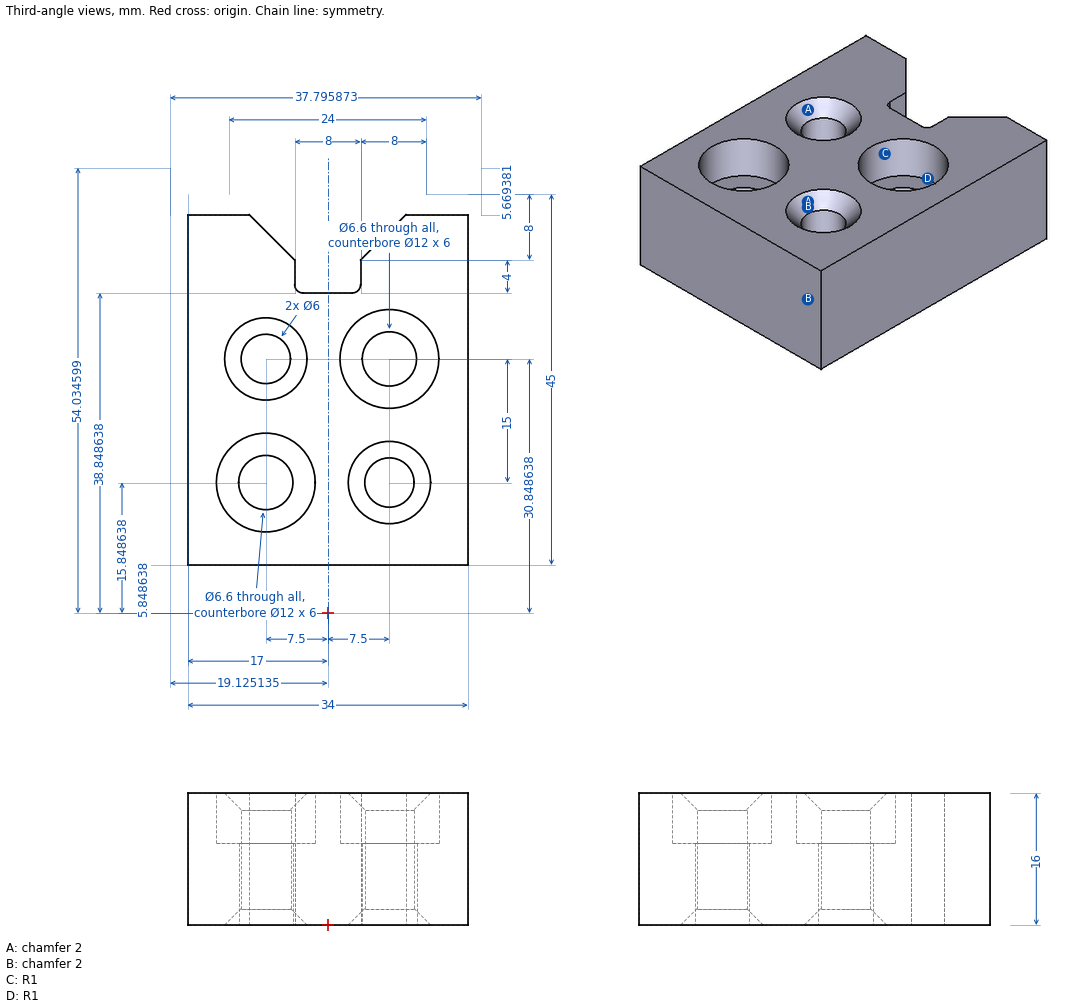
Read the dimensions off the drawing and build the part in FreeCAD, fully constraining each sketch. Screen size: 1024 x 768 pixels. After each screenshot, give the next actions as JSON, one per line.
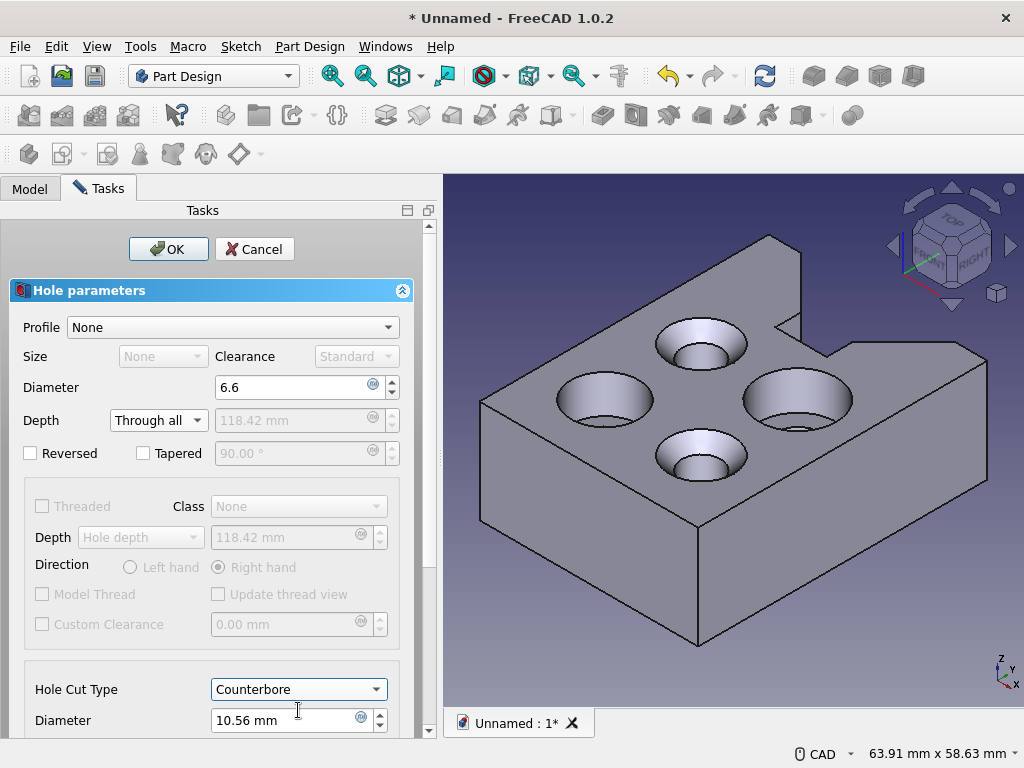
{"action": "triple_click", "coordinate": [292, 720]}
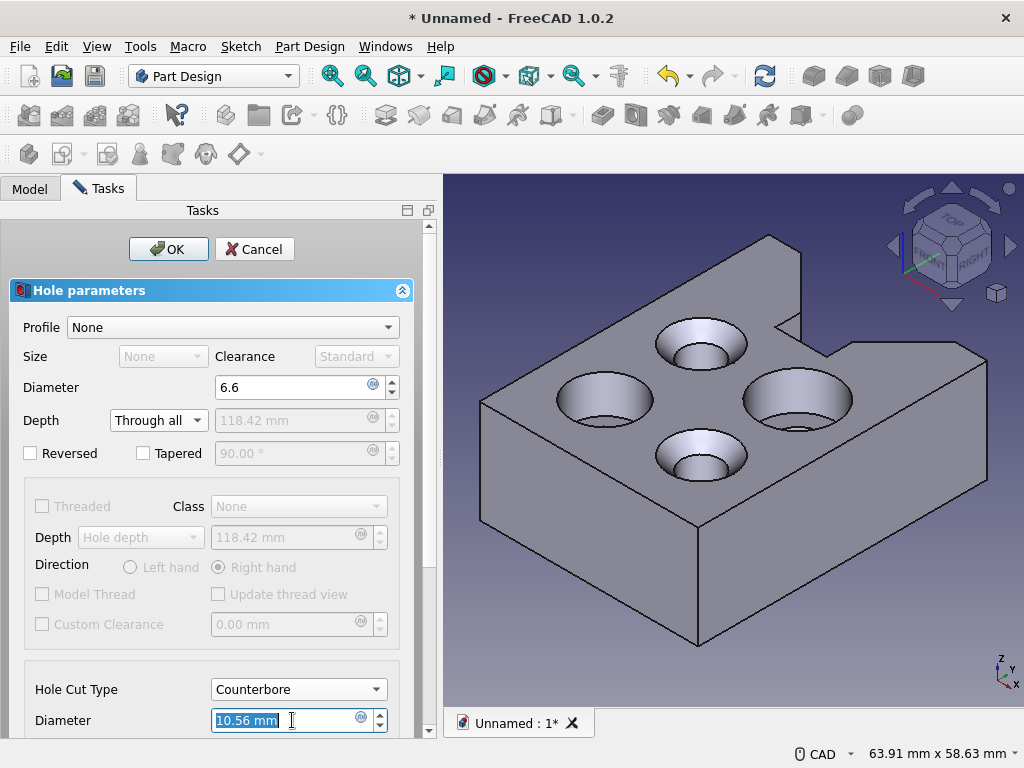
{"action": "type", "text": "12"}
{"action": "key", "text": "Tab"}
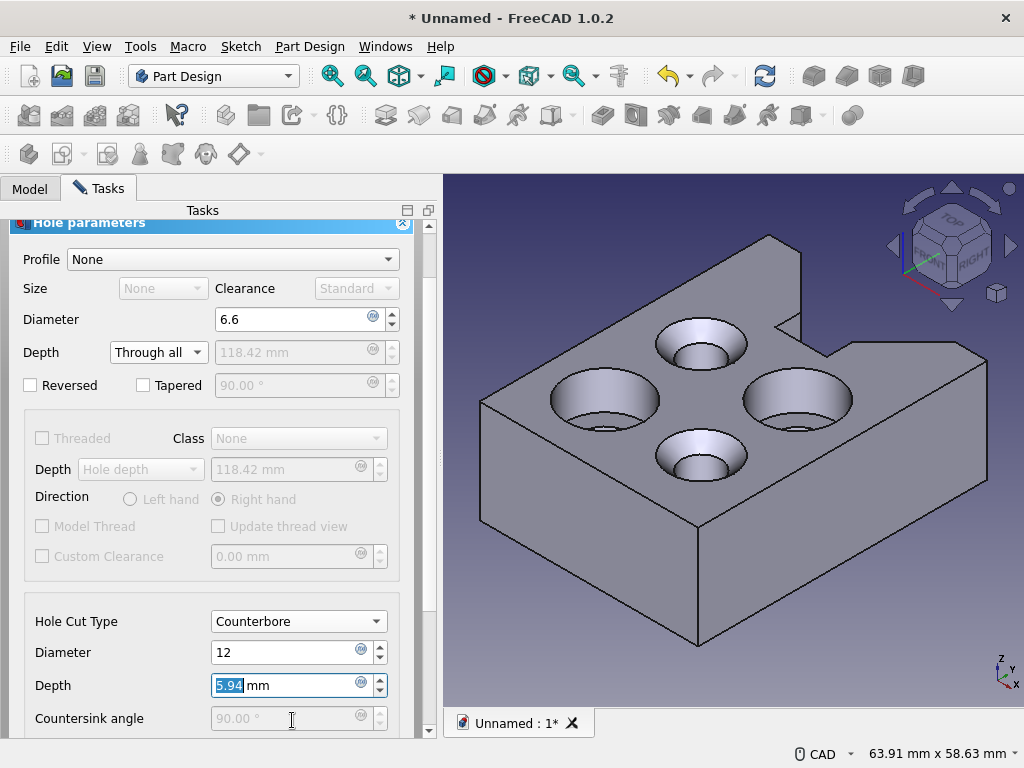
{"action": "type", "text": "6"}
{"action": "key", "text": "Tab"}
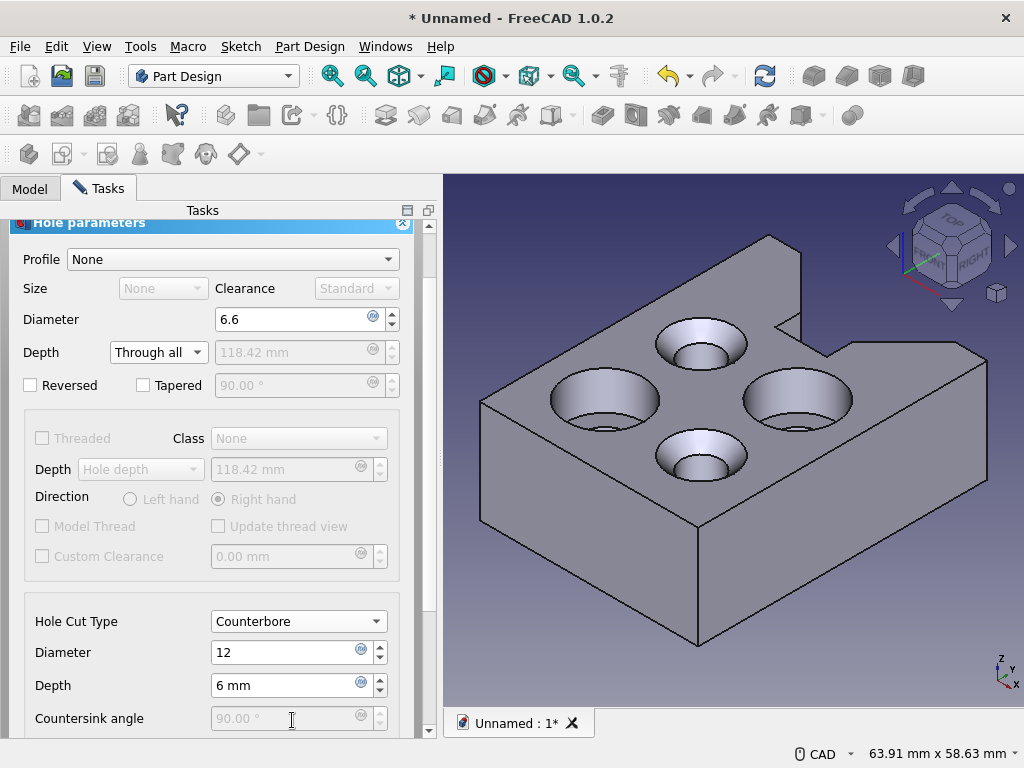
{"action": "scroll", "coordinate": [429, 479], "scroll_direction": "up", "scroll_amount": 2}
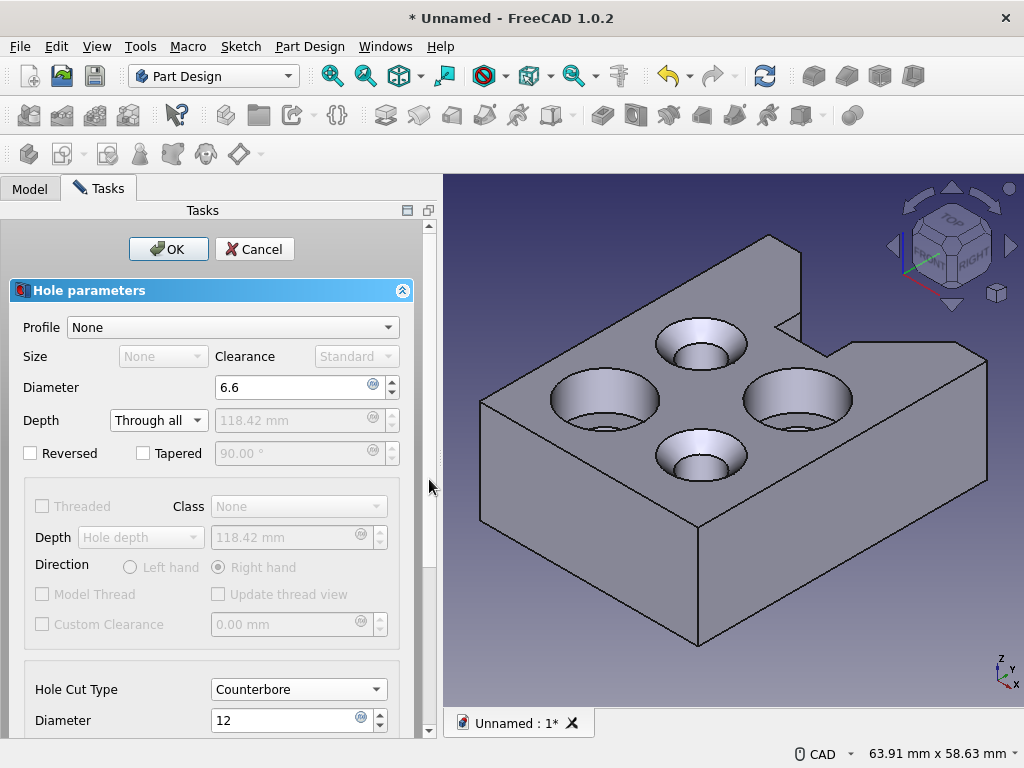
{"action": "left_click", "coordinate": [169, 249]}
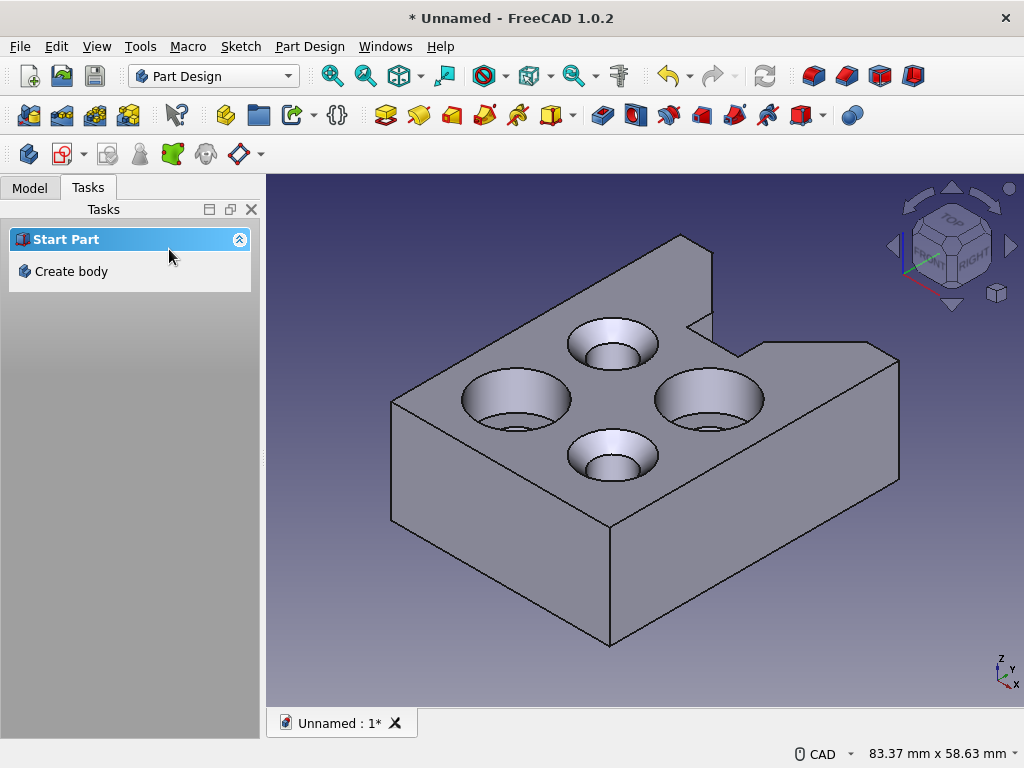
{"action": "key", "text": "2"}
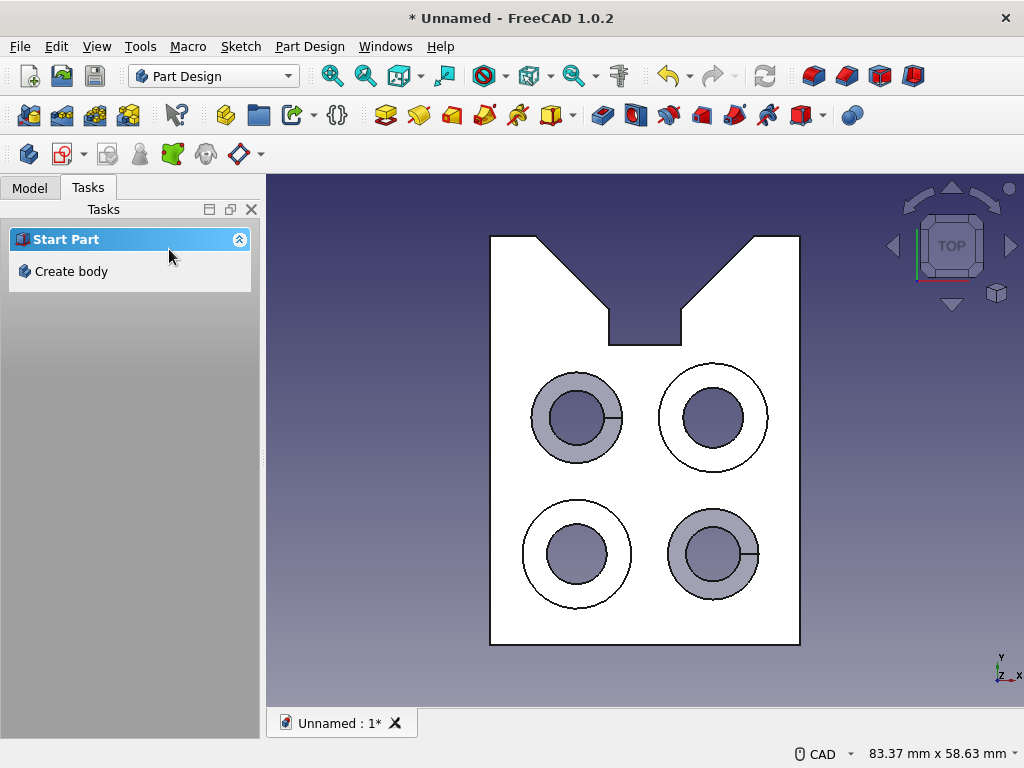
{"action": "key", "text": "0"}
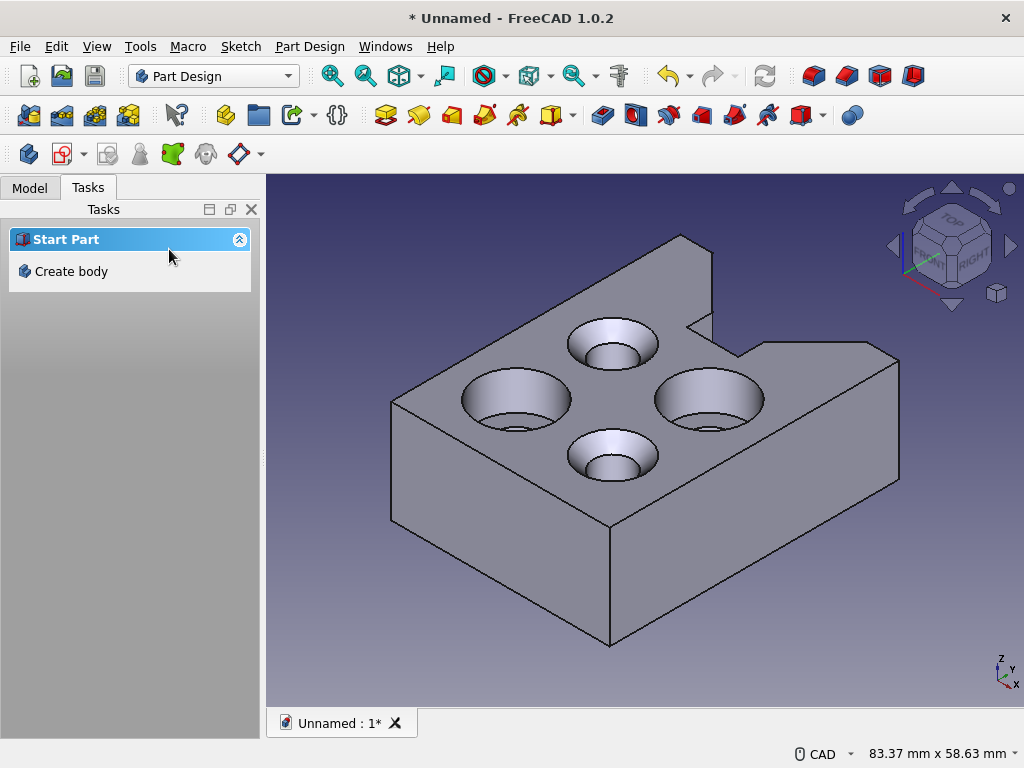
{"action": "key", "text": "1"}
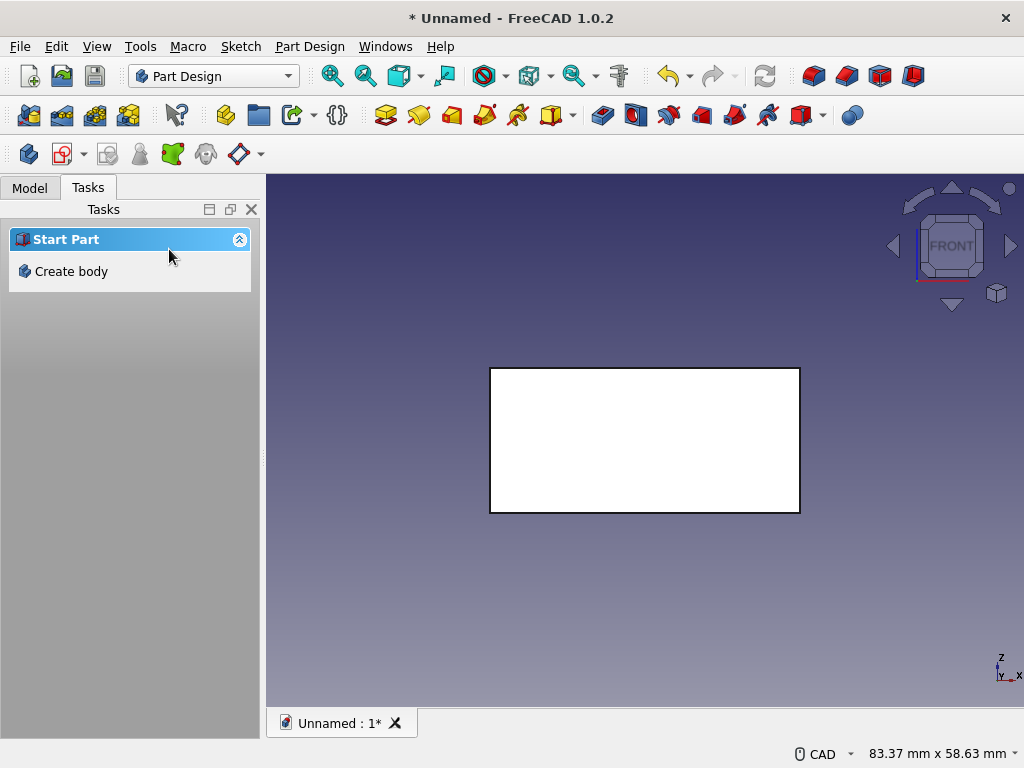
{"action": "left_click", "coordinate": [333, 76]}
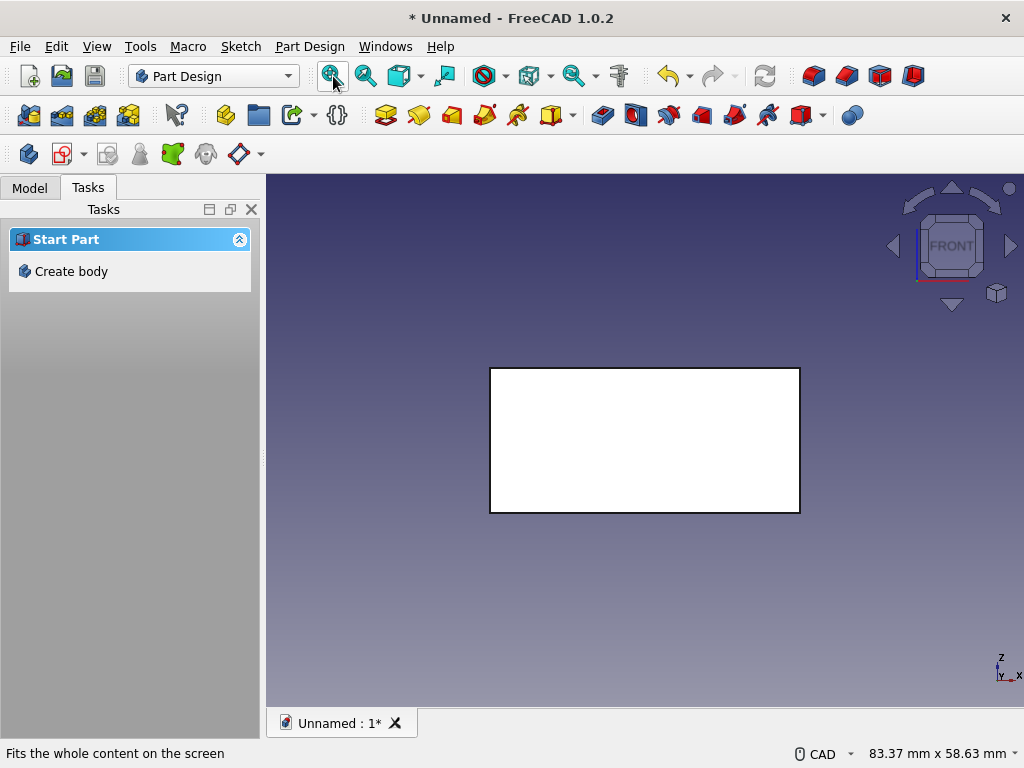
{"action": "key", "text": "3"}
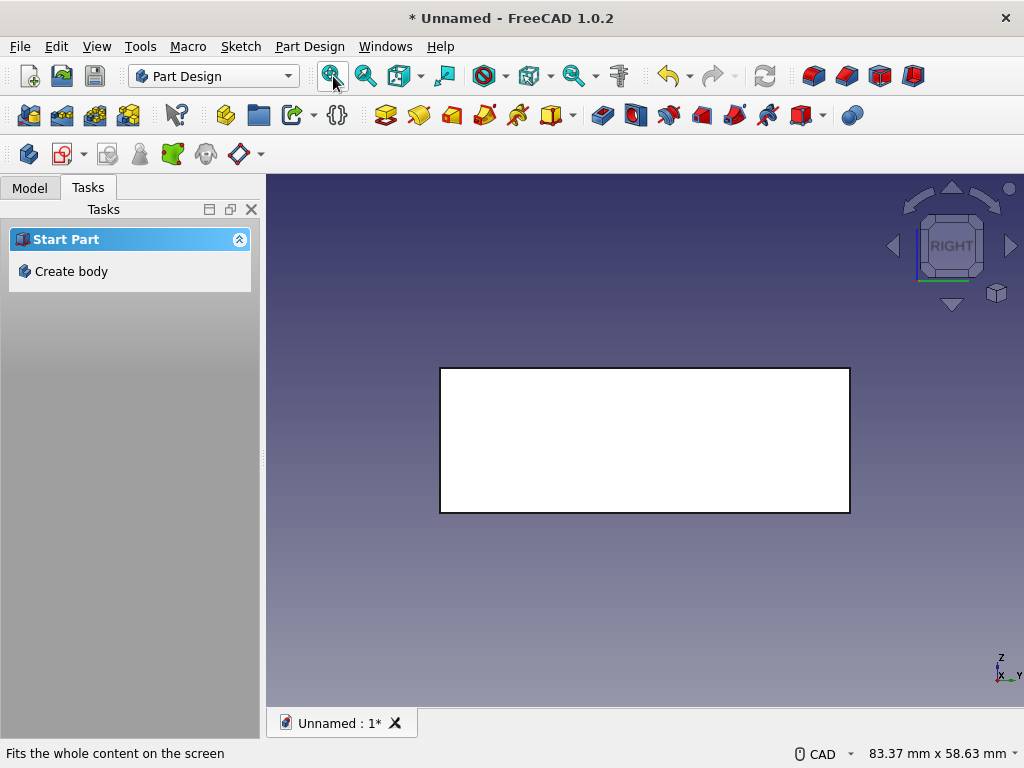
{"action": "key", "text": "5"}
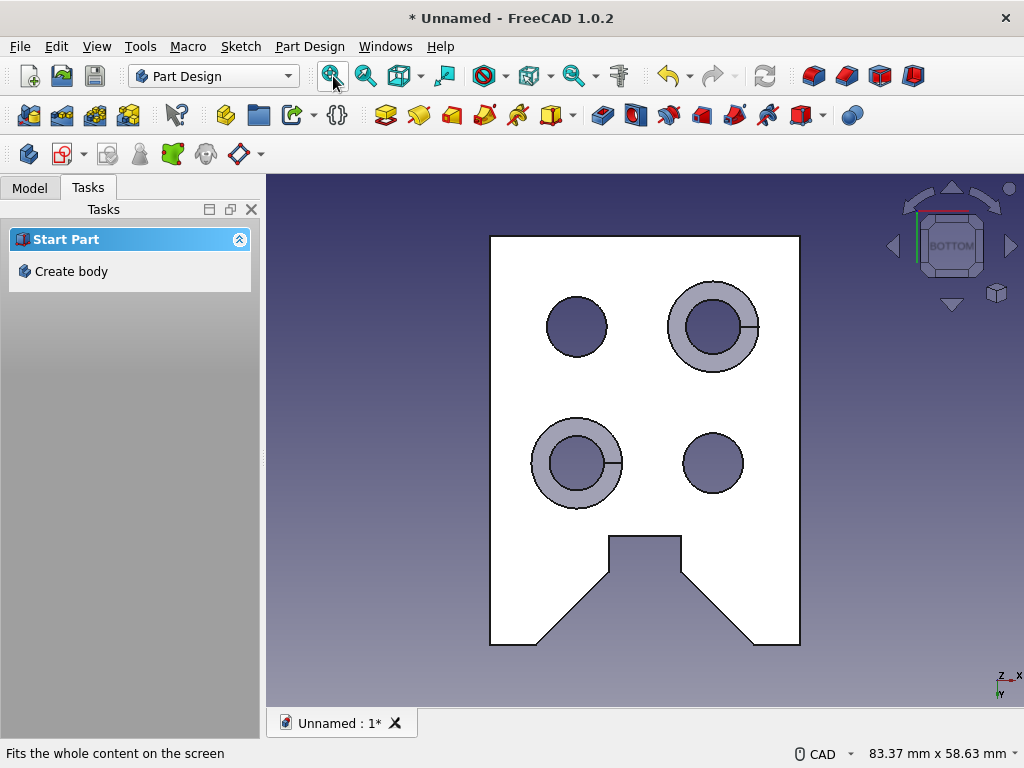
{"action": "key", "text": "4"}